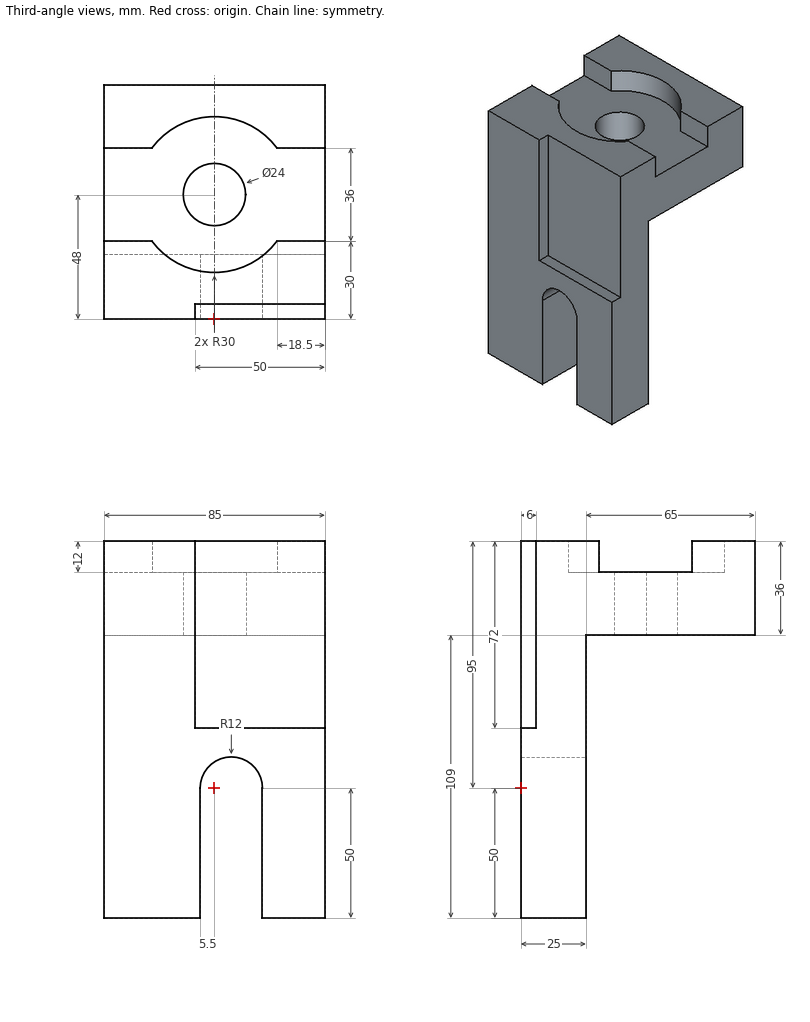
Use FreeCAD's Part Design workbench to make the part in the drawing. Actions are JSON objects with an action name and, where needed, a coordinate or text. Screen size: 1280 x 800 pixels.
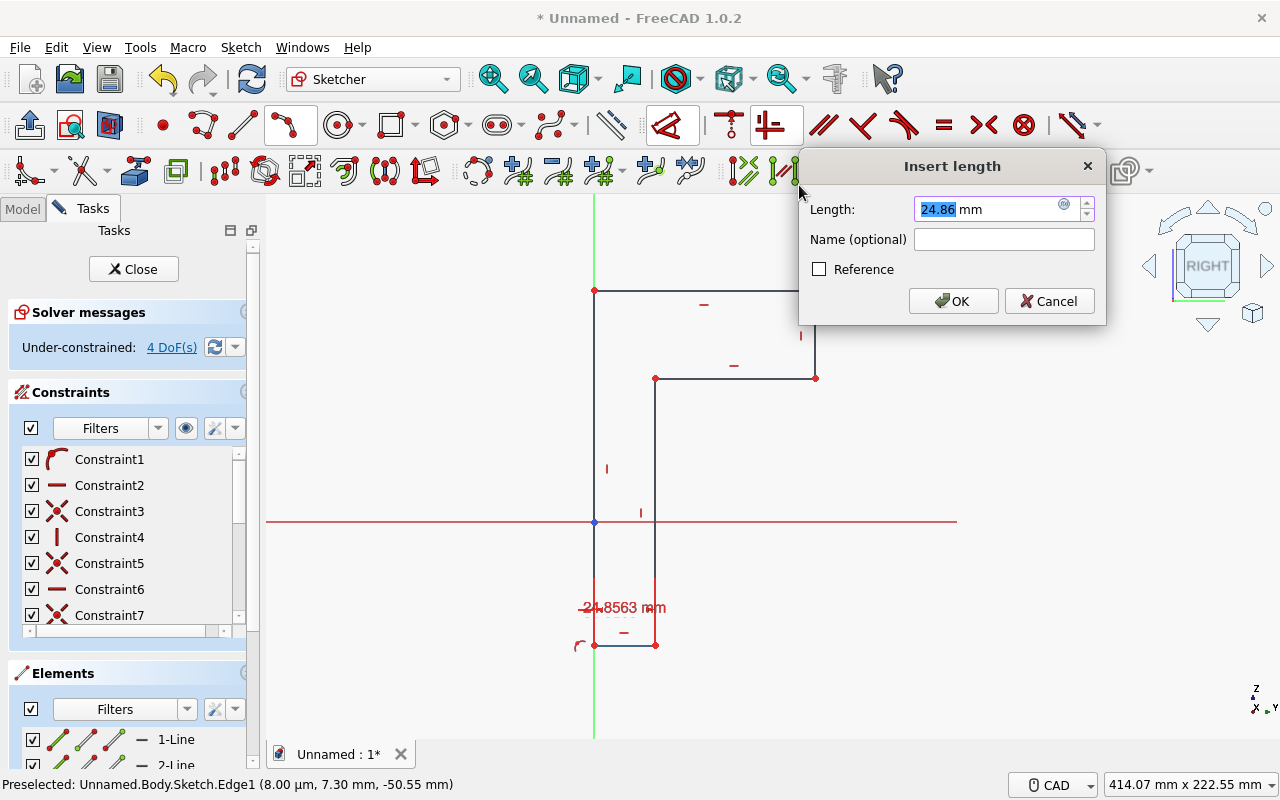
{"action": "type", "text": "25"}
{"action": "key", "text": "Return"}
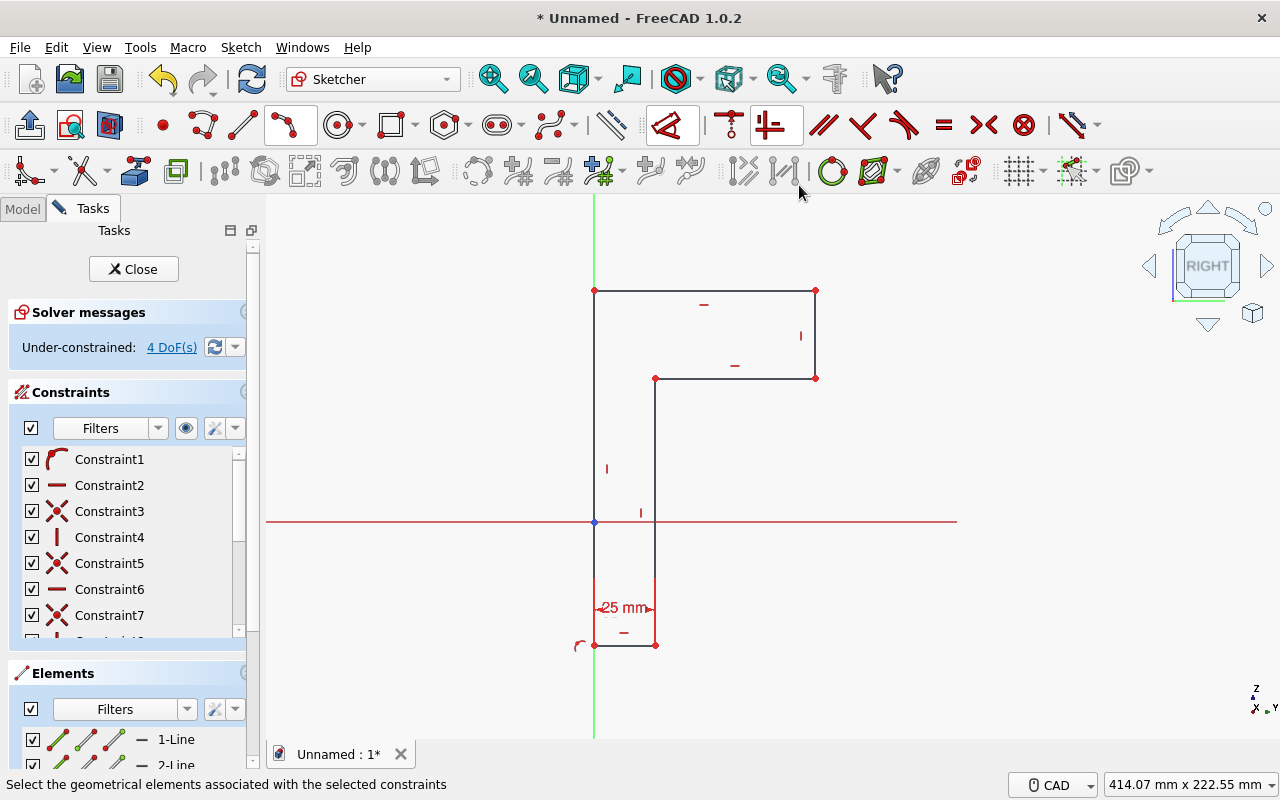
{"action": "left_click", "coordinate": [703, 379]}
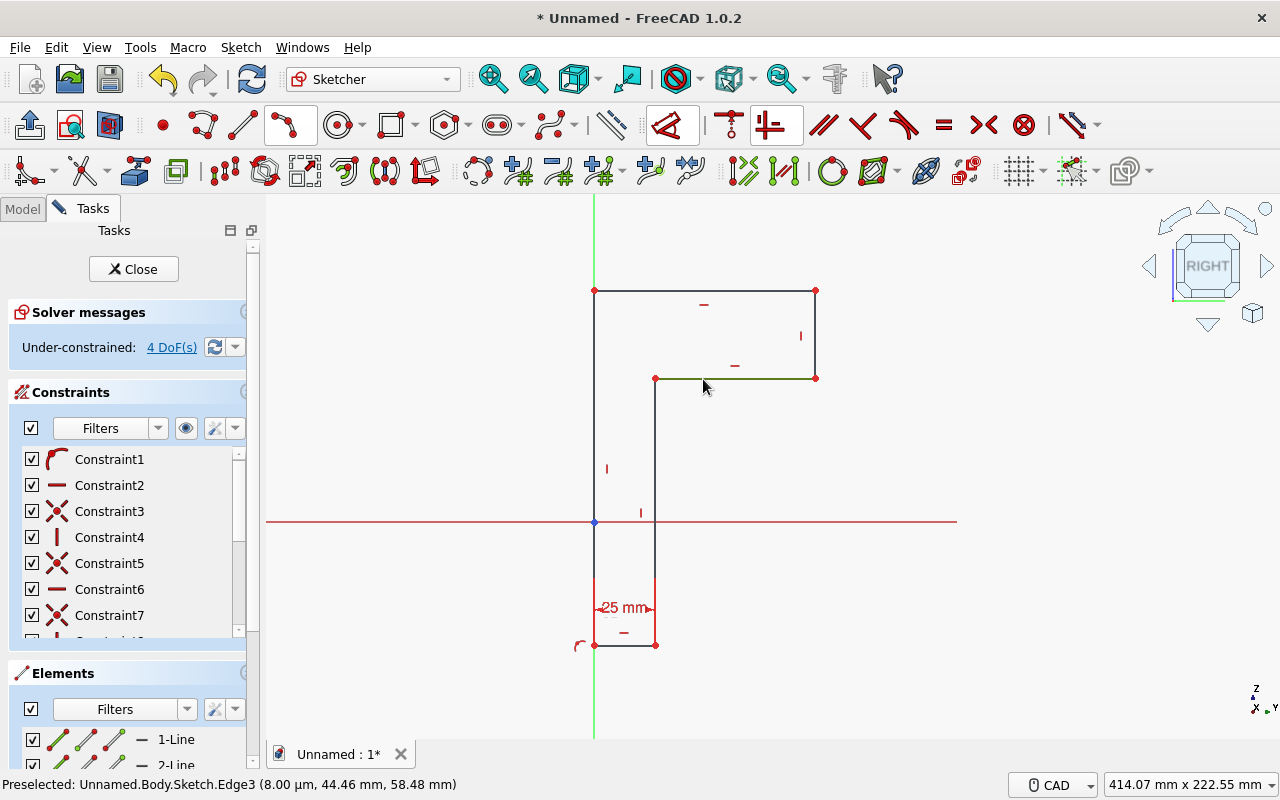
{"action": "left_click", "coordinate": [694, 126]}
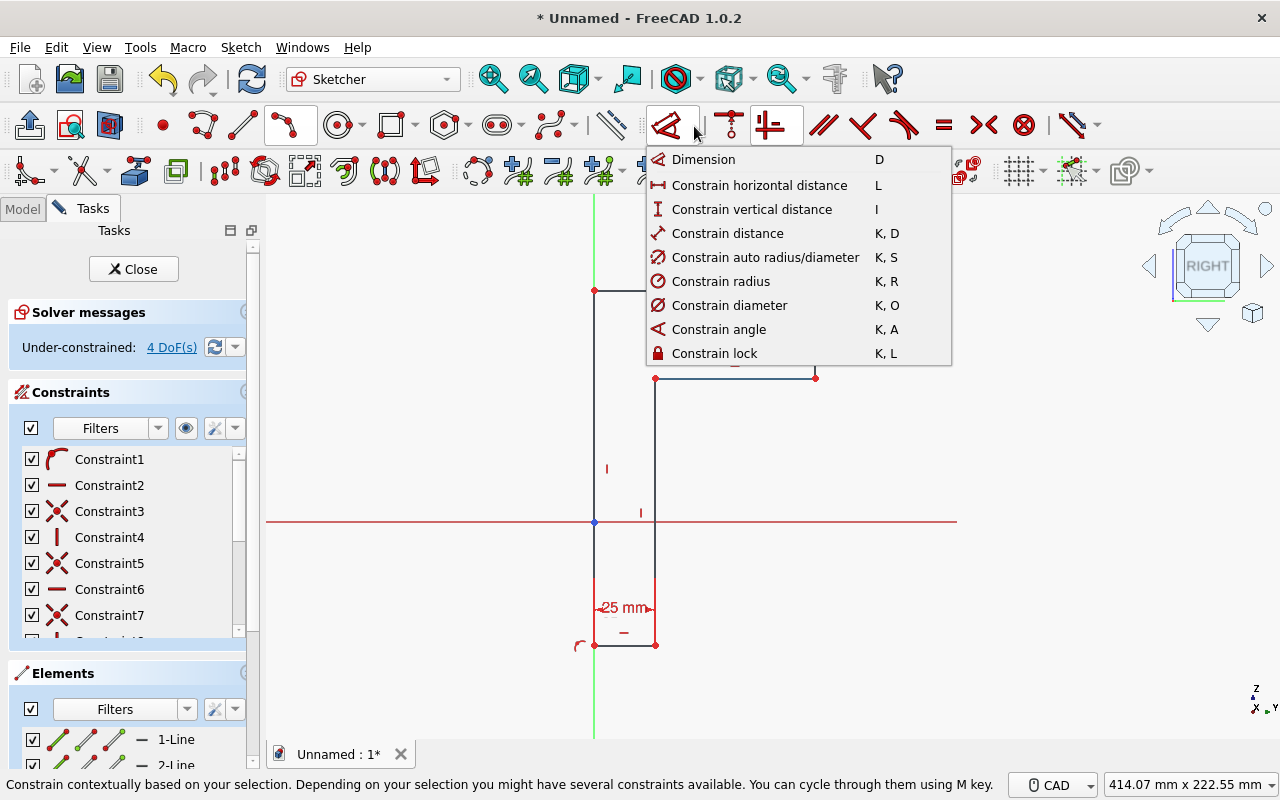
{"action": "left_click", "coordinate": [799, 185]}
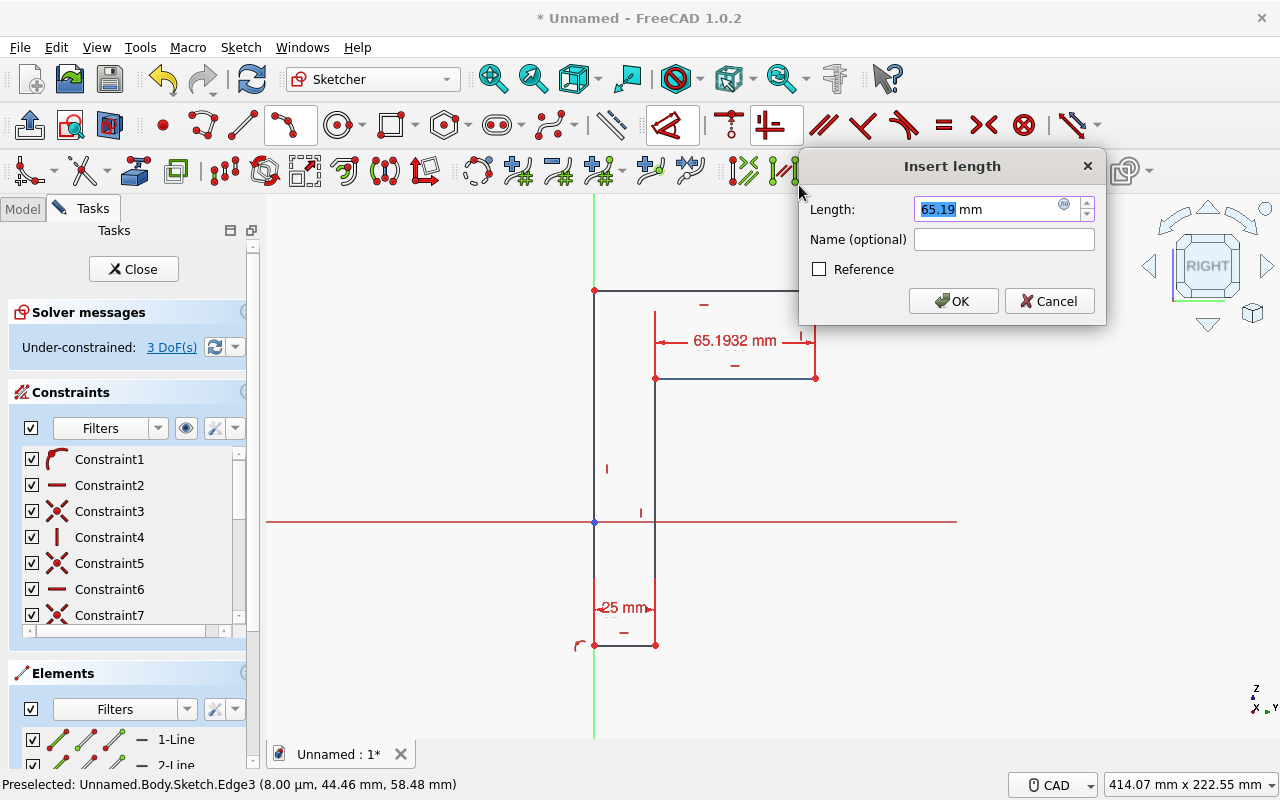
{"action": "type", "text": "65"}
{"action": "key", "text": "Return"}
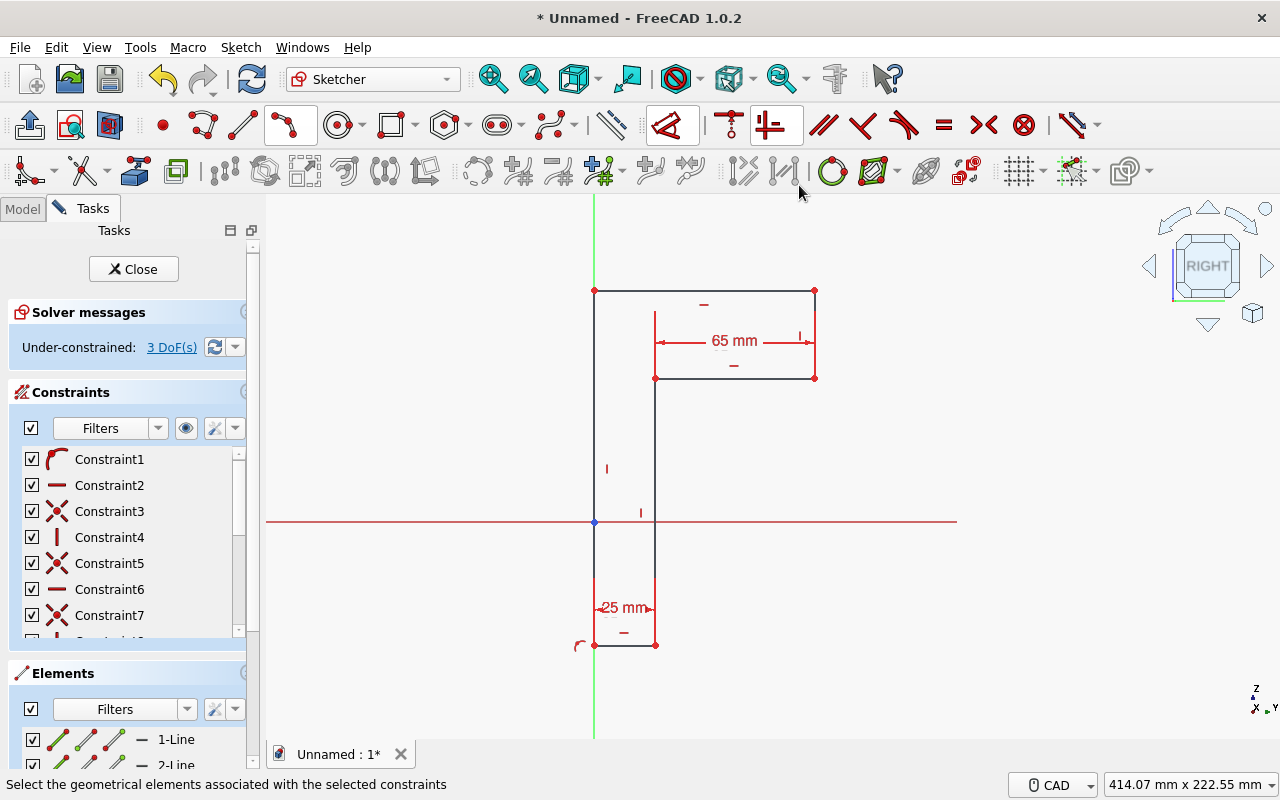
{"action": "left_click", "coordinate": [815, 353]}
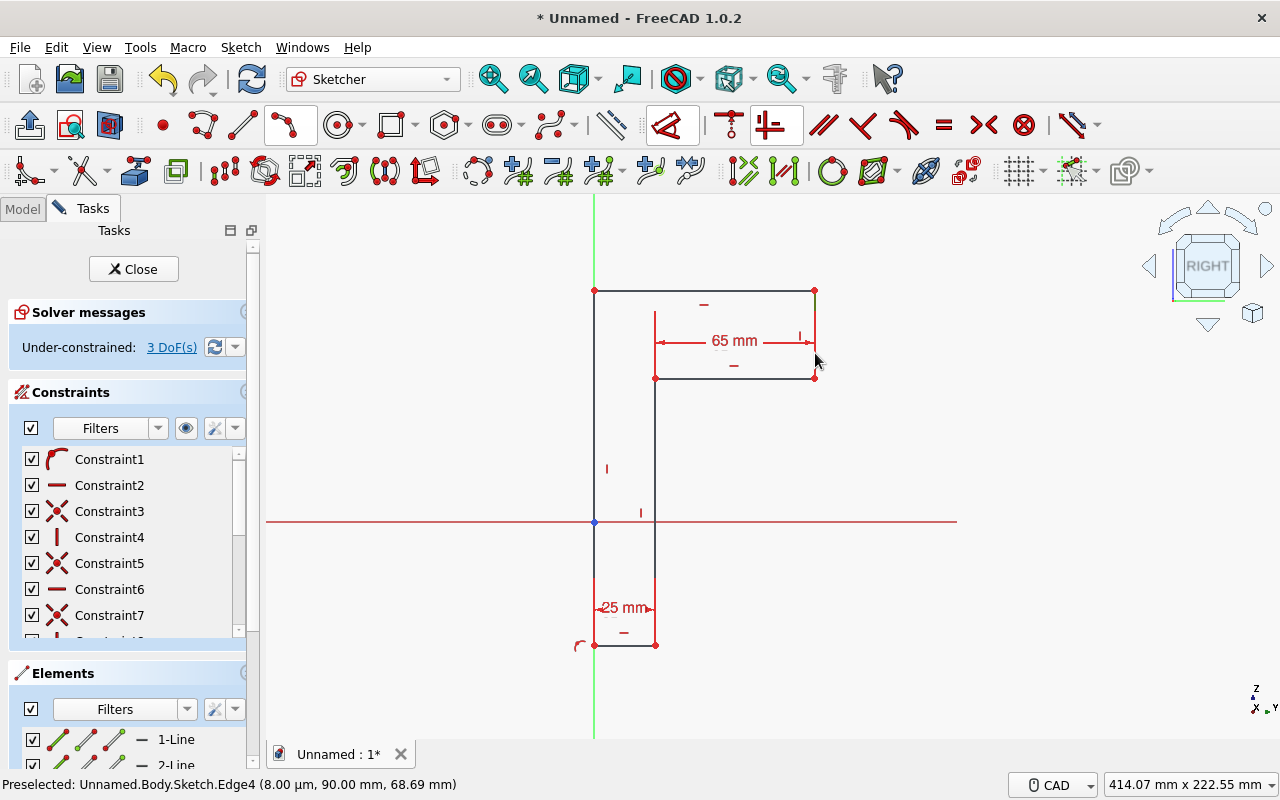
{"action": "left_click", "coordinate": [694, 126]}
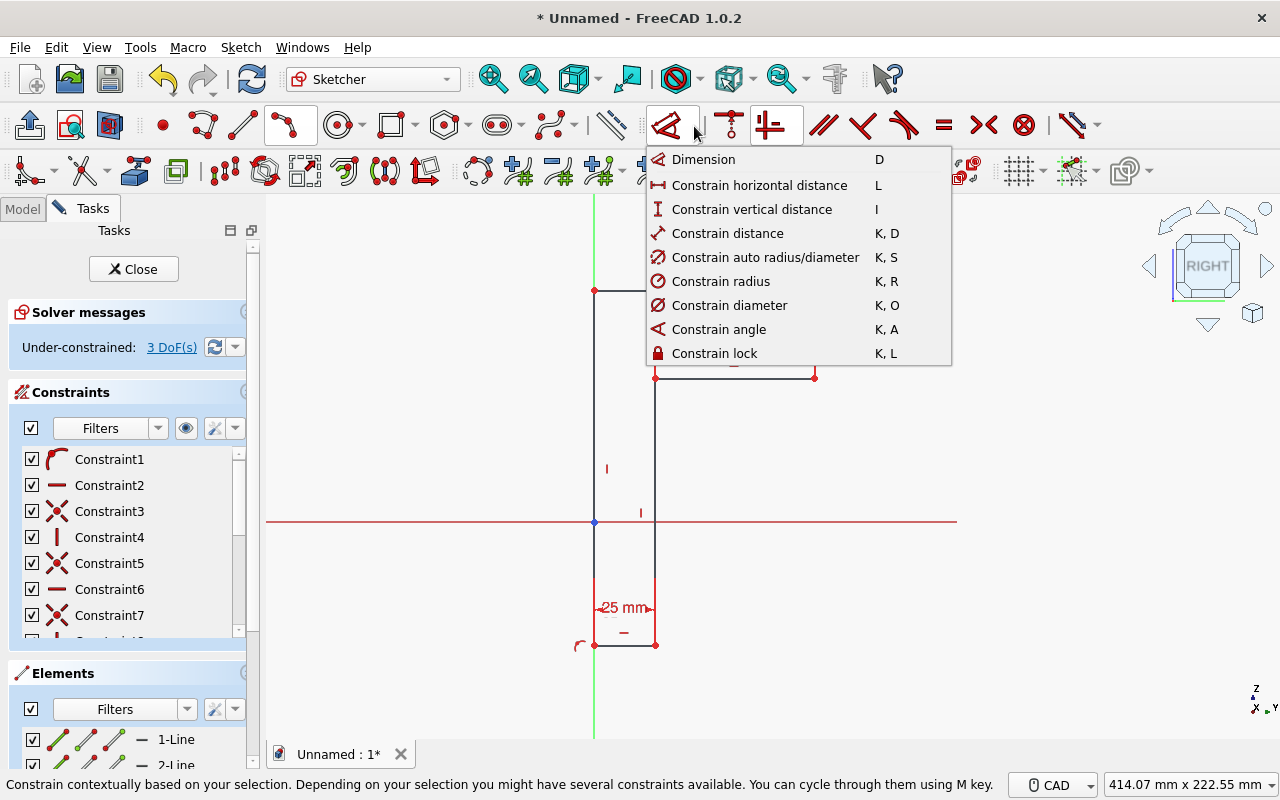
{"action": "left_click", "coordinate": [799, 209]}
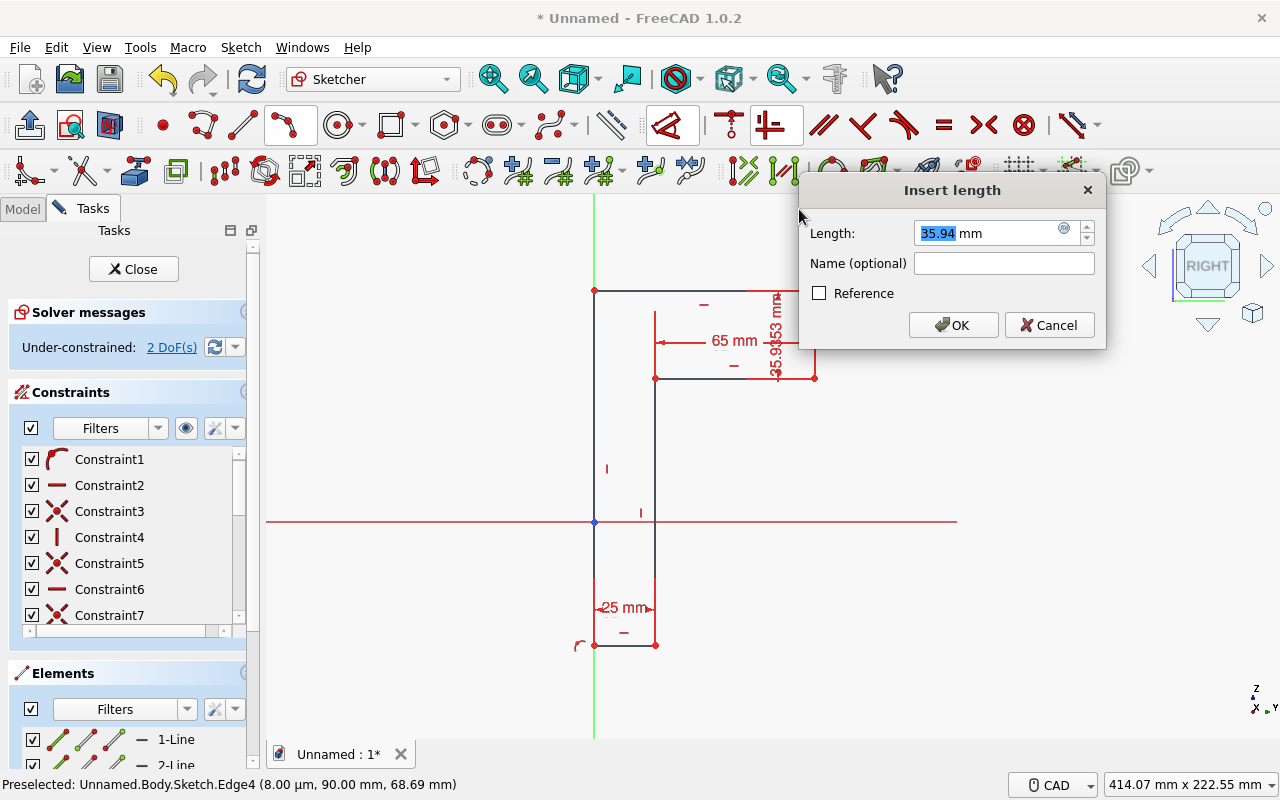
{"action": "type", "text": "36"}
{"action": "key", "text": "Return"}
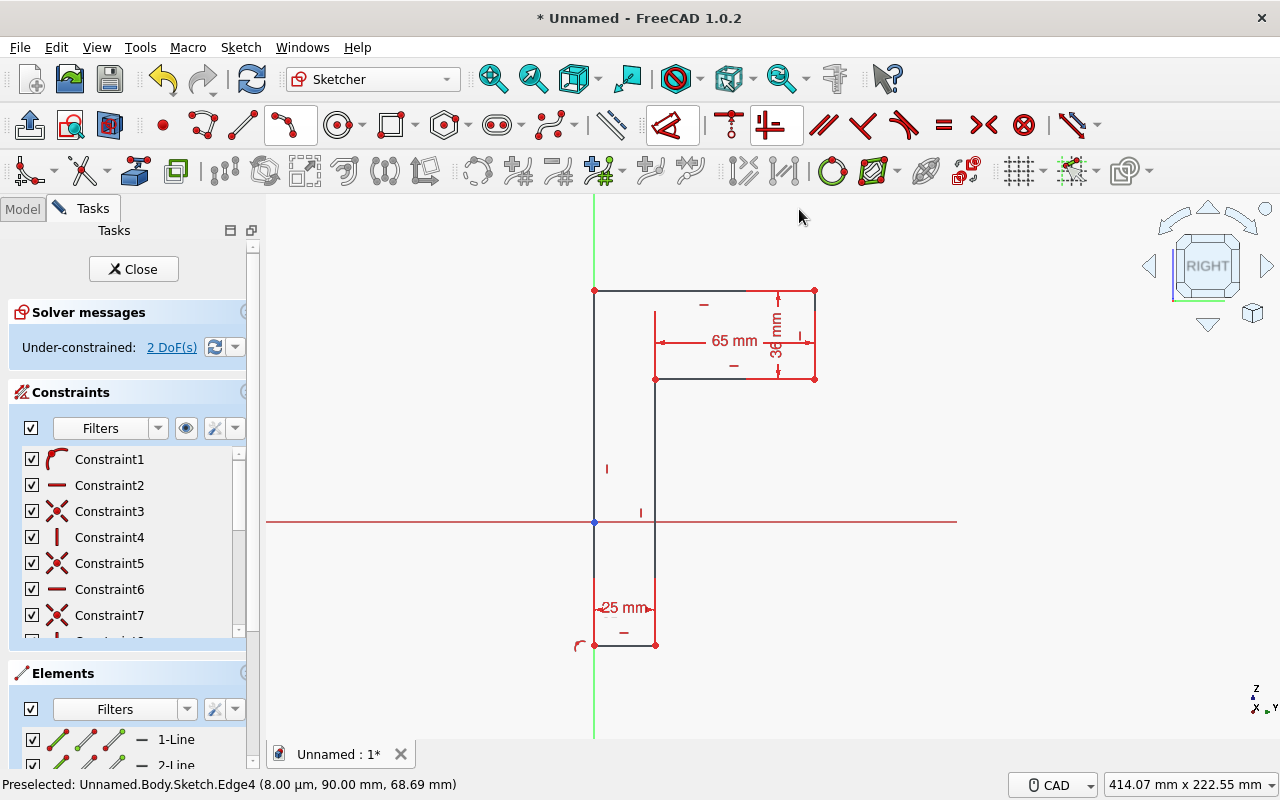
{"action": "left_click", "coordinate": [655, 566]}